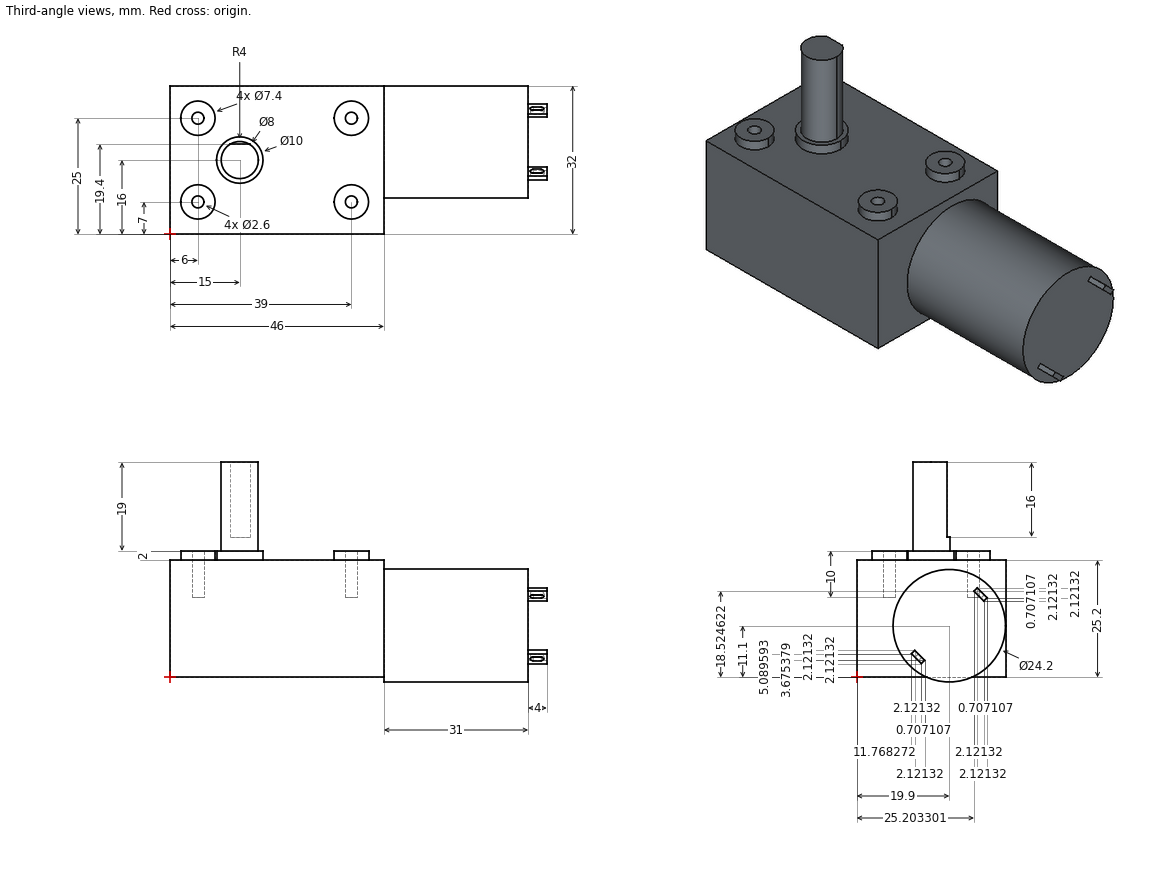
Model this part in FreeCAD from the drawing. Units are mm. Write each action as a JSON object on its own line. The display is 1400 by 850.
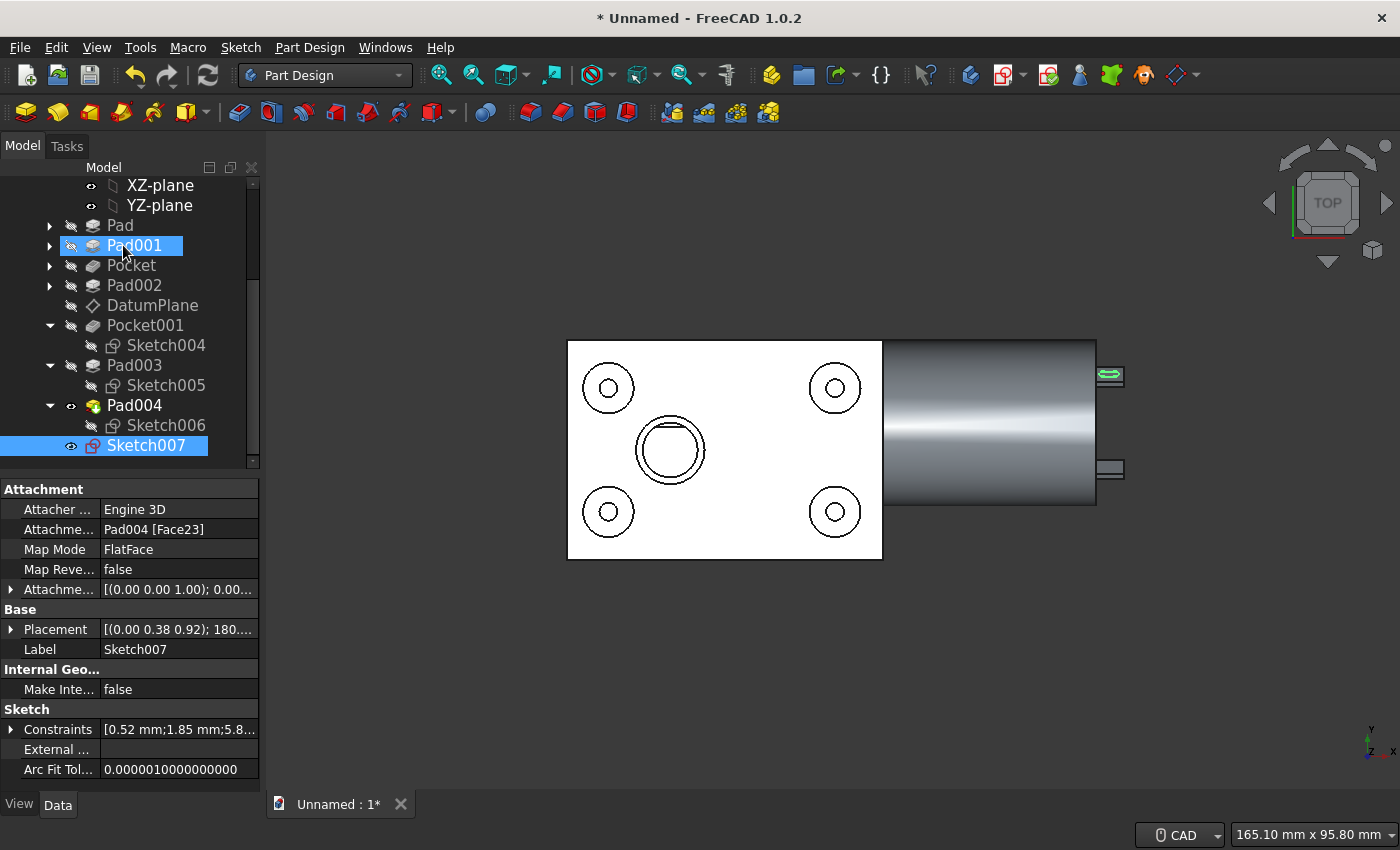
{"action": "left_click", "coordinate": [240, 112]}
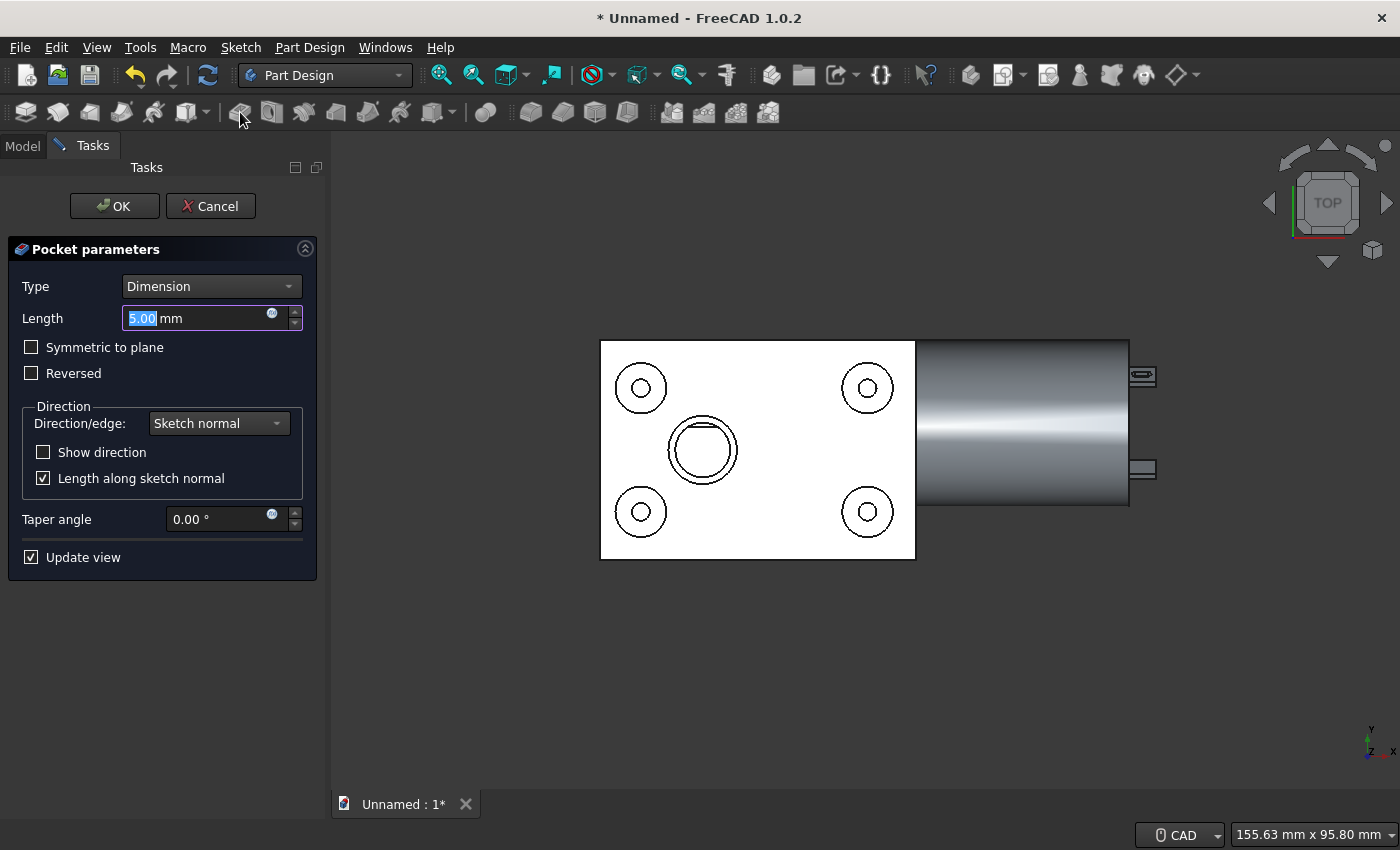
{"action": "left_click", "coordinate": [212, 286]}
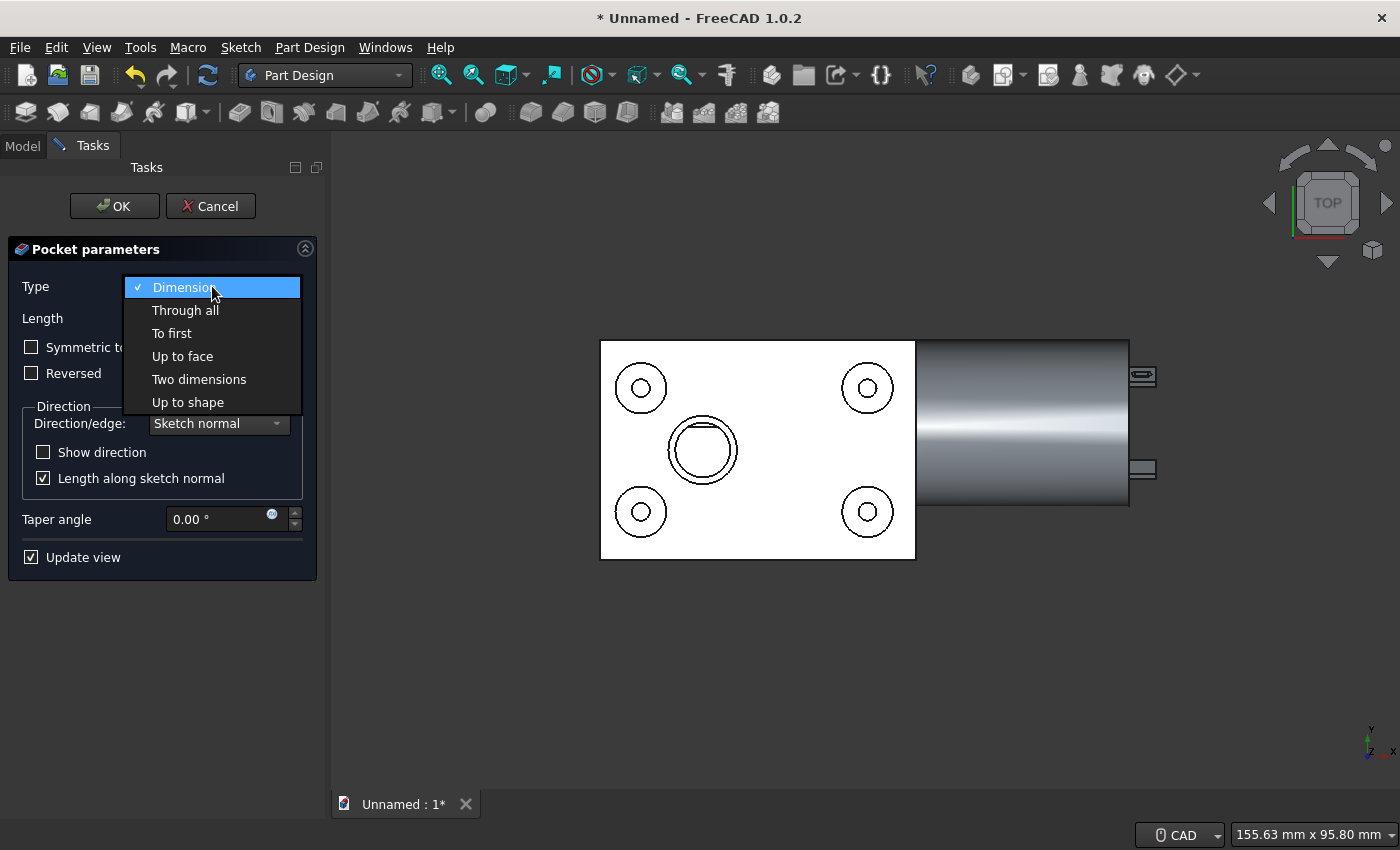
{"action": "left_click", "coordinate": [212, 310]}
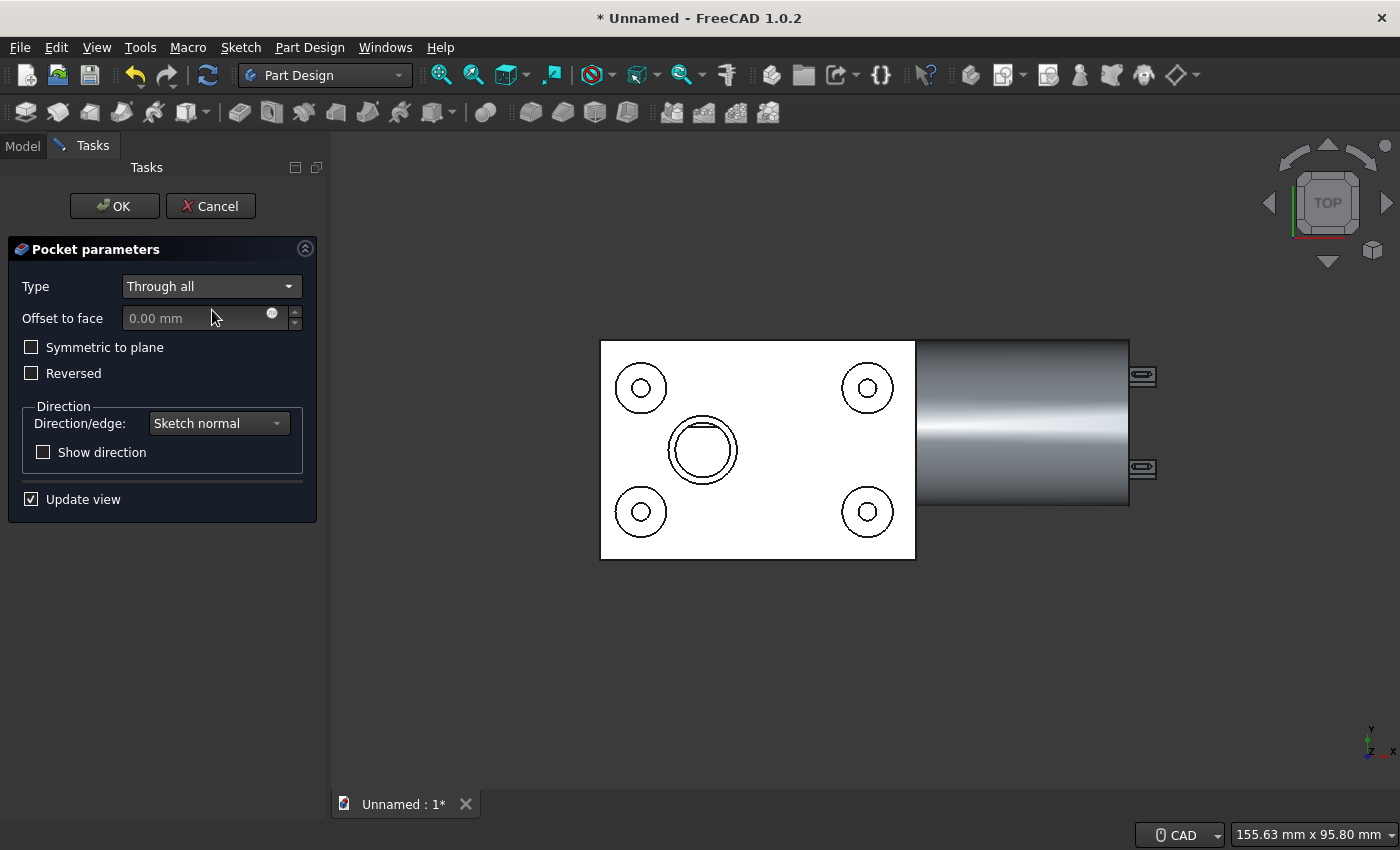
{"action": "left_click", "coordinate": [115, 206]}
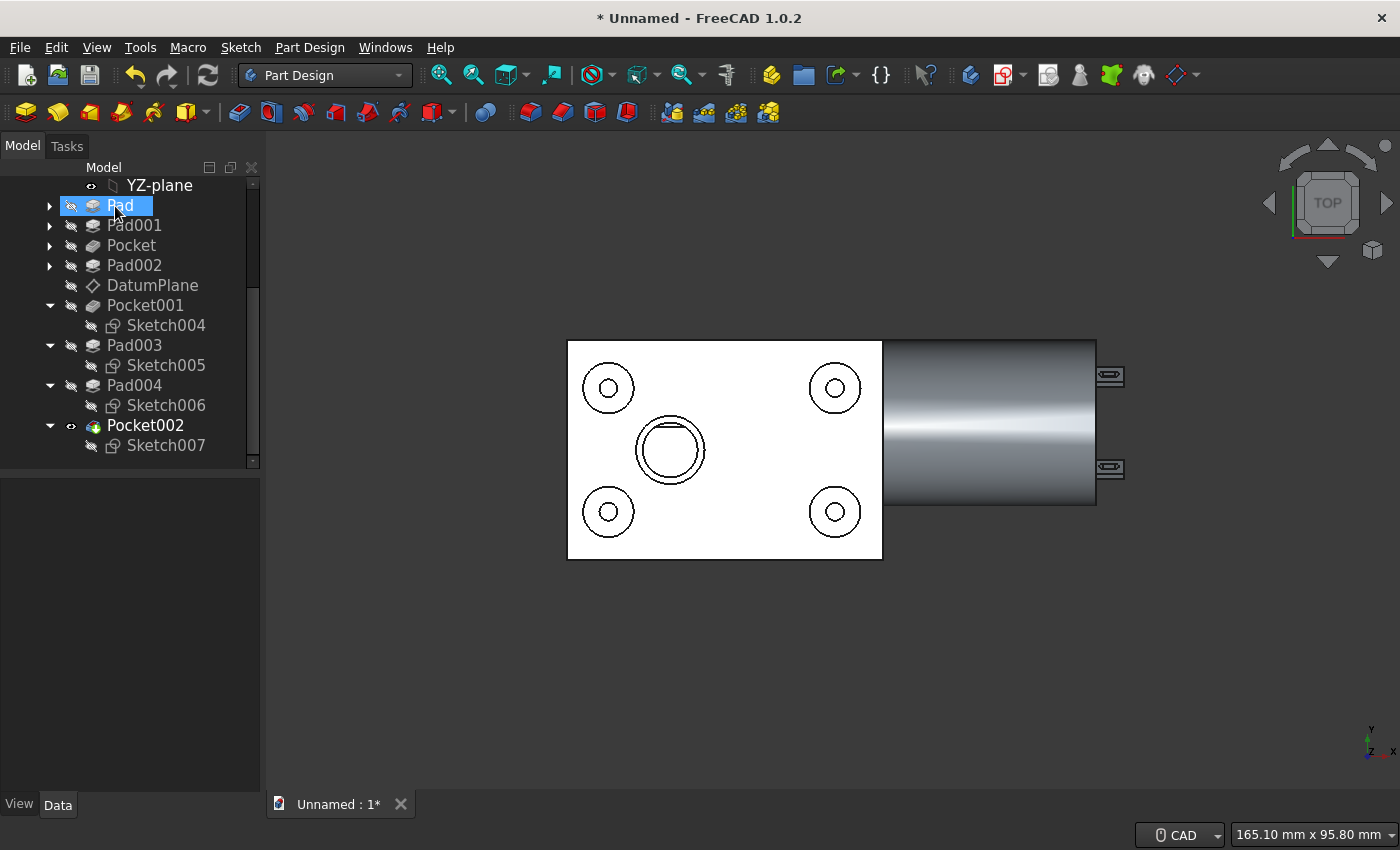
{"action": "key", "text": "0"}